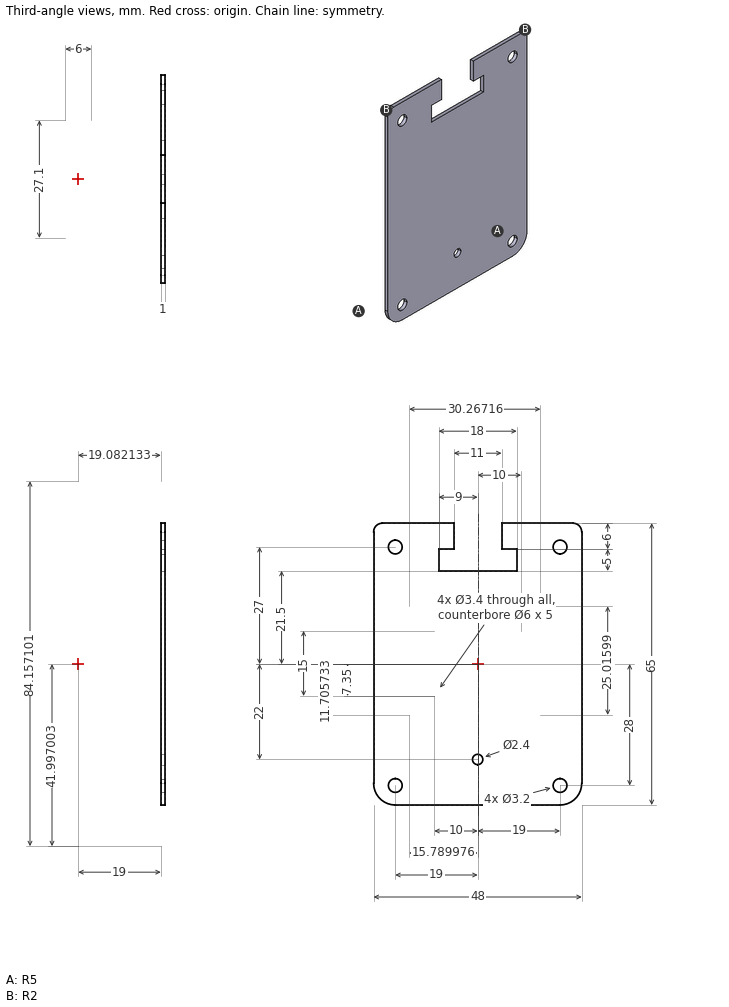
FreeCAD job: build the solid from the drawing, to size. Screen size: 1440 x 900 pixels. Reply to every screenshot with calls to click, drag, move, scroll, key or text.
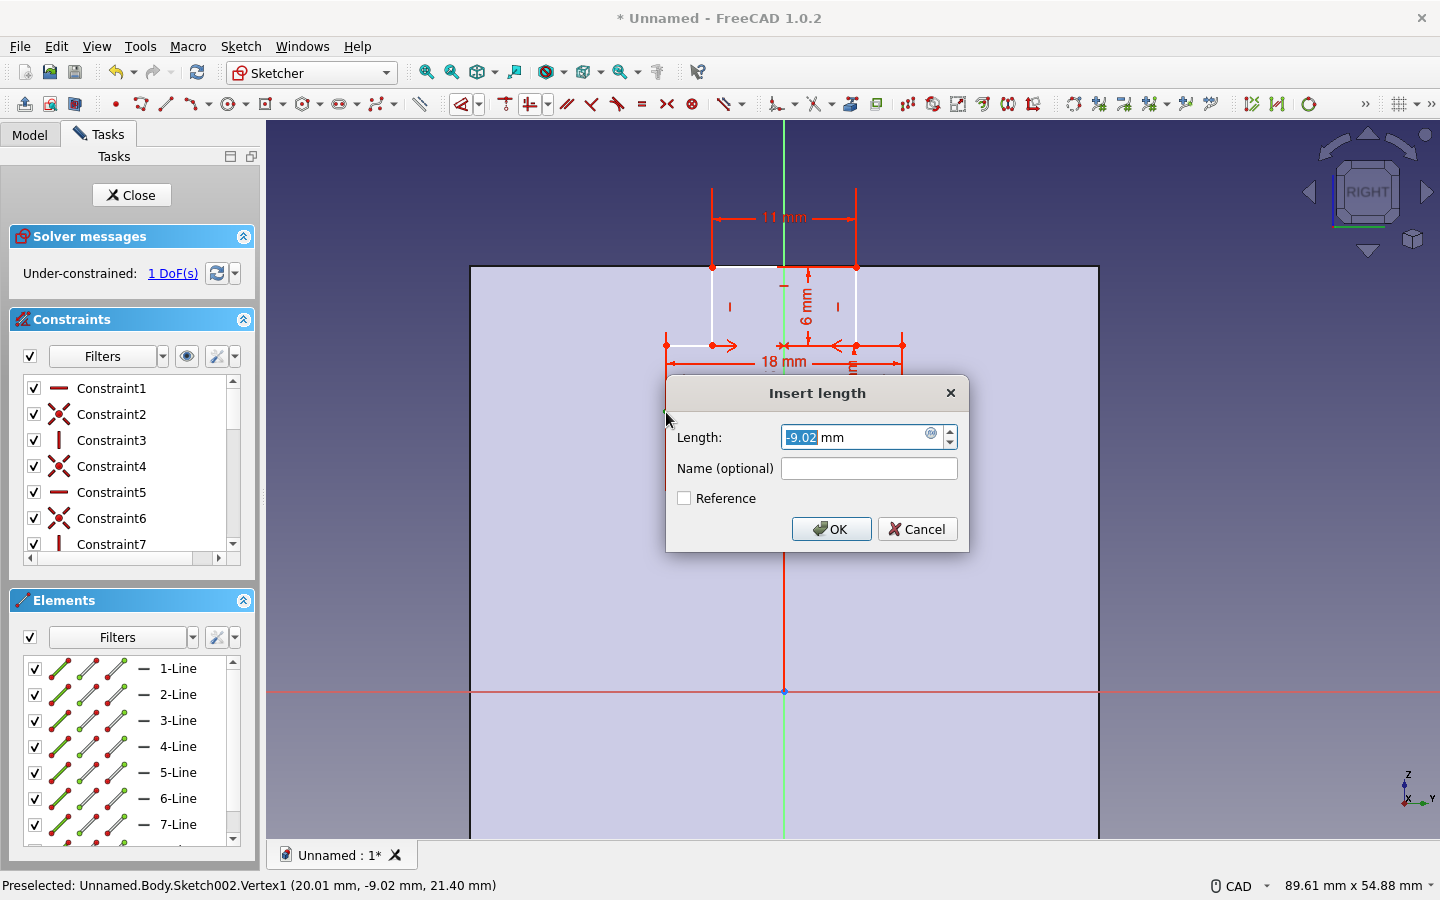
text(-9)
key(Return)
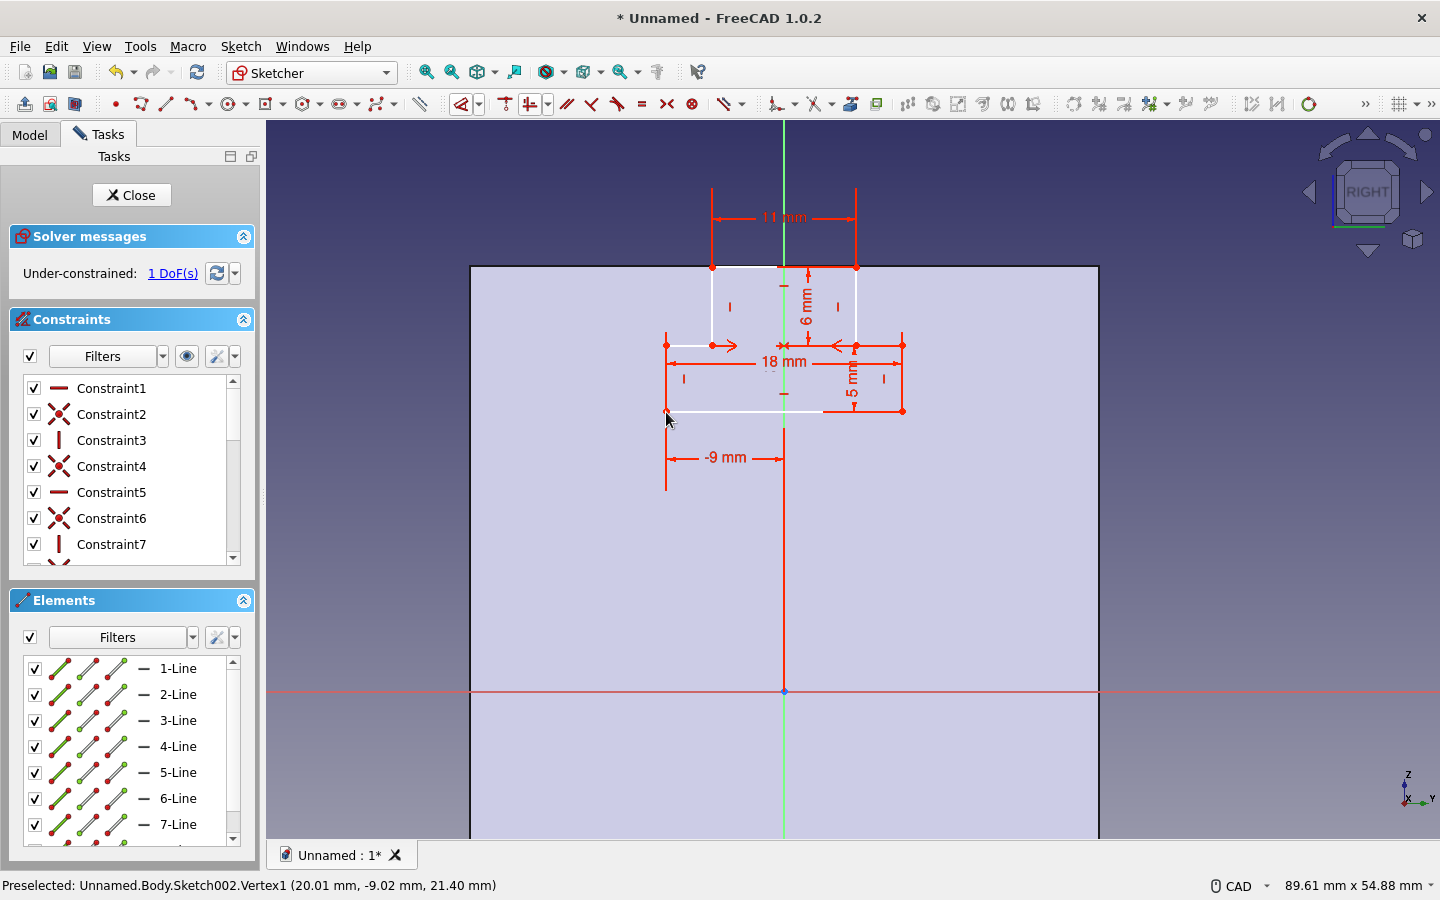
click(666, 412)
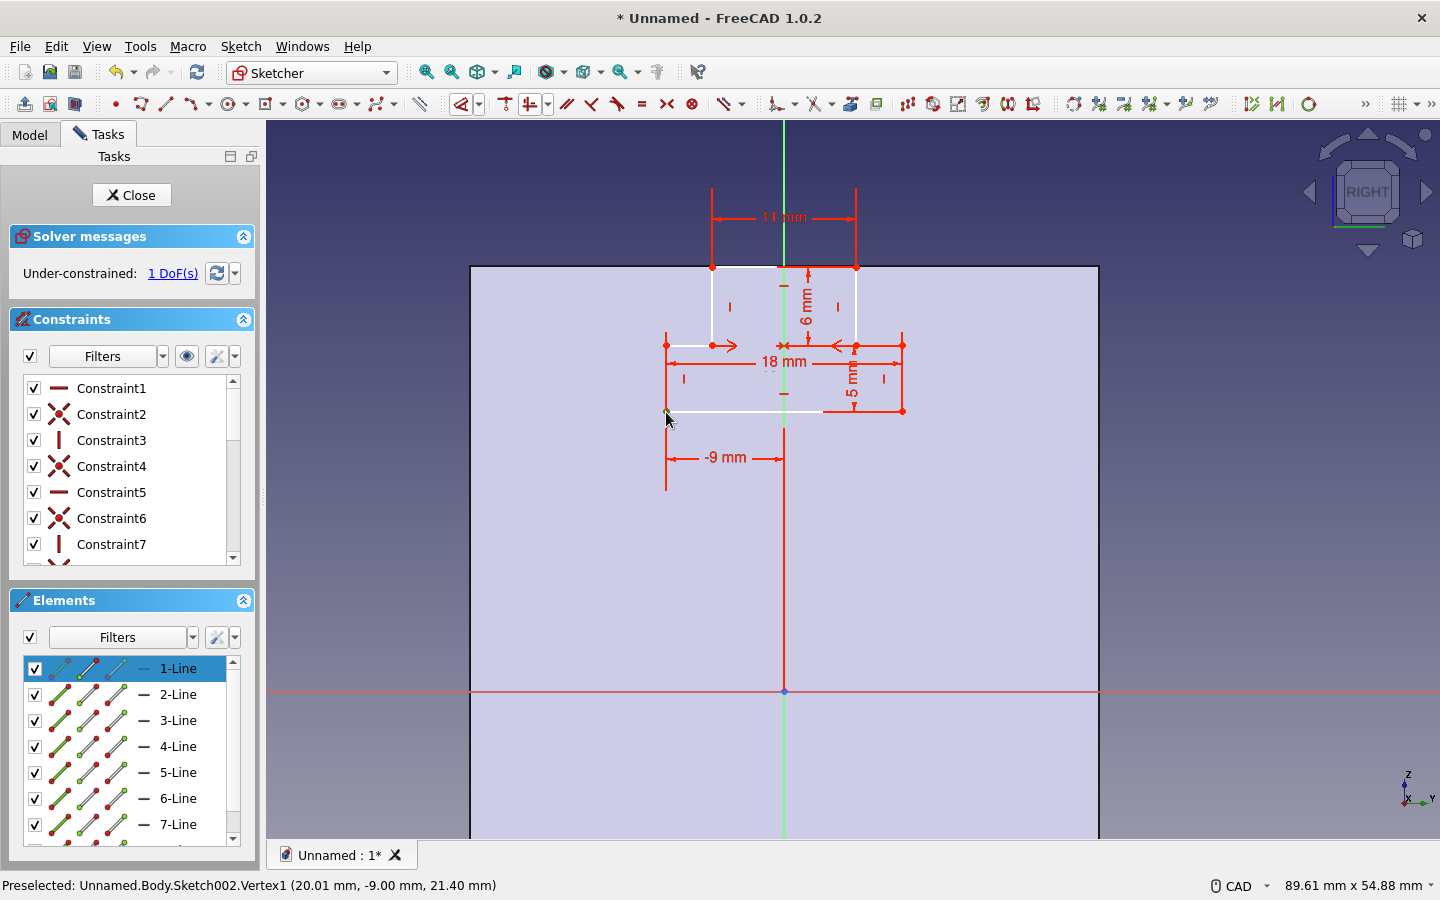
key(i)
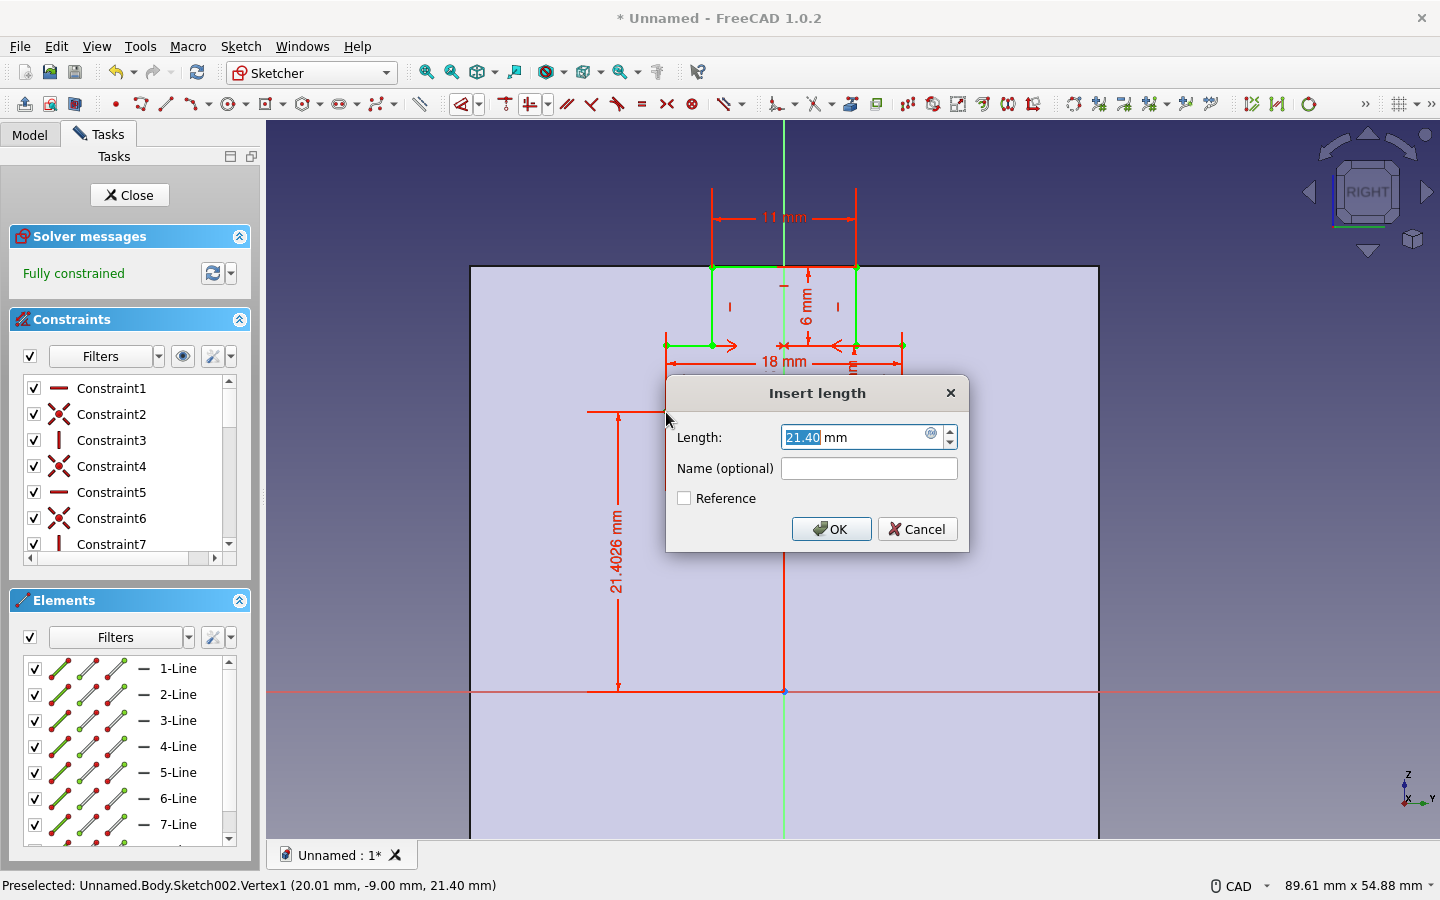
text(21.5)
key(Return)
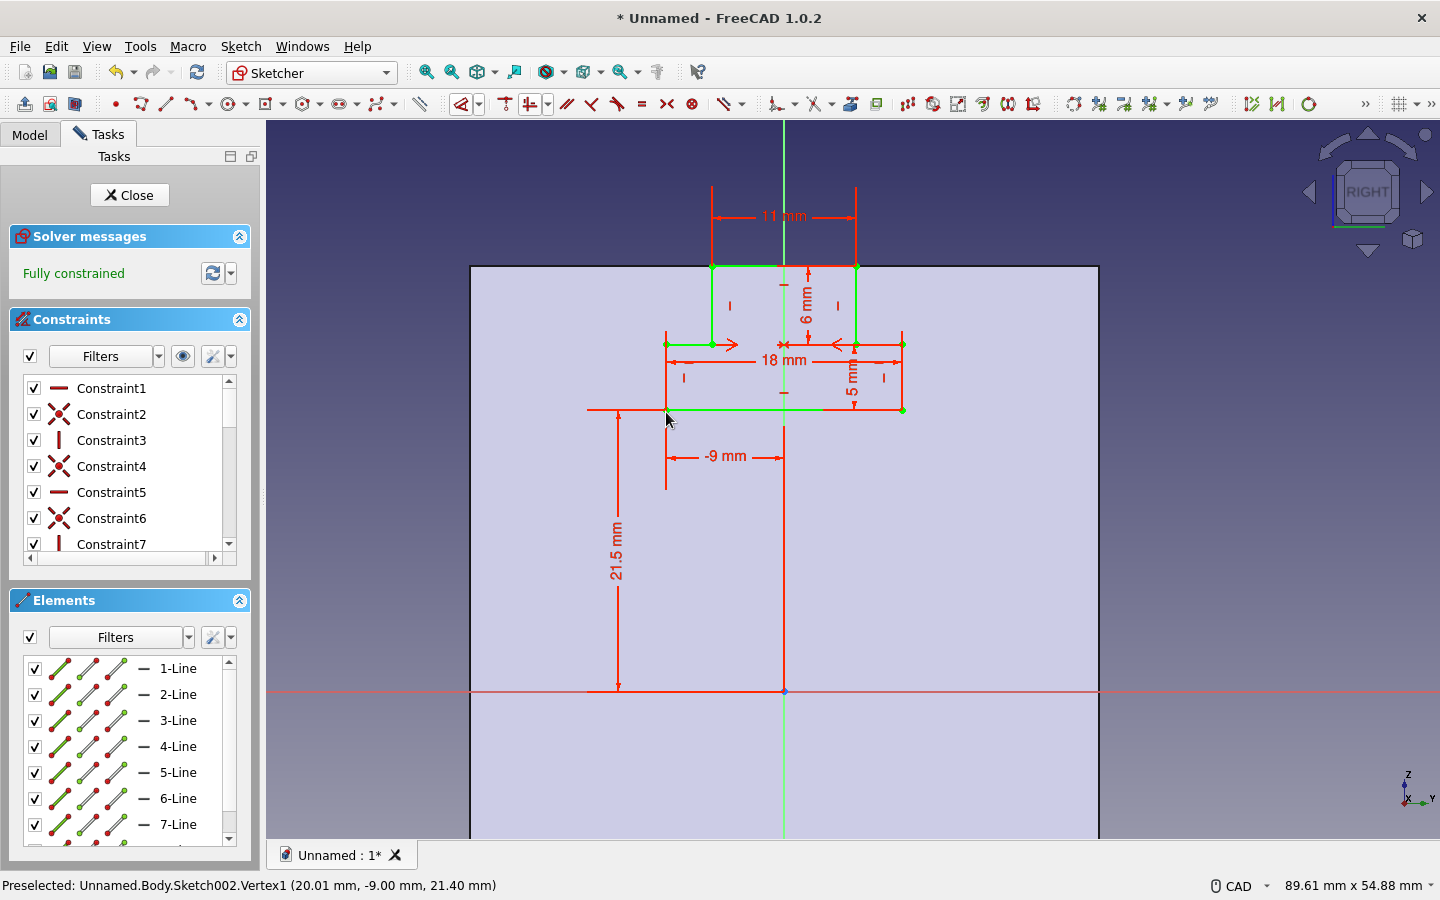
click(130, 195)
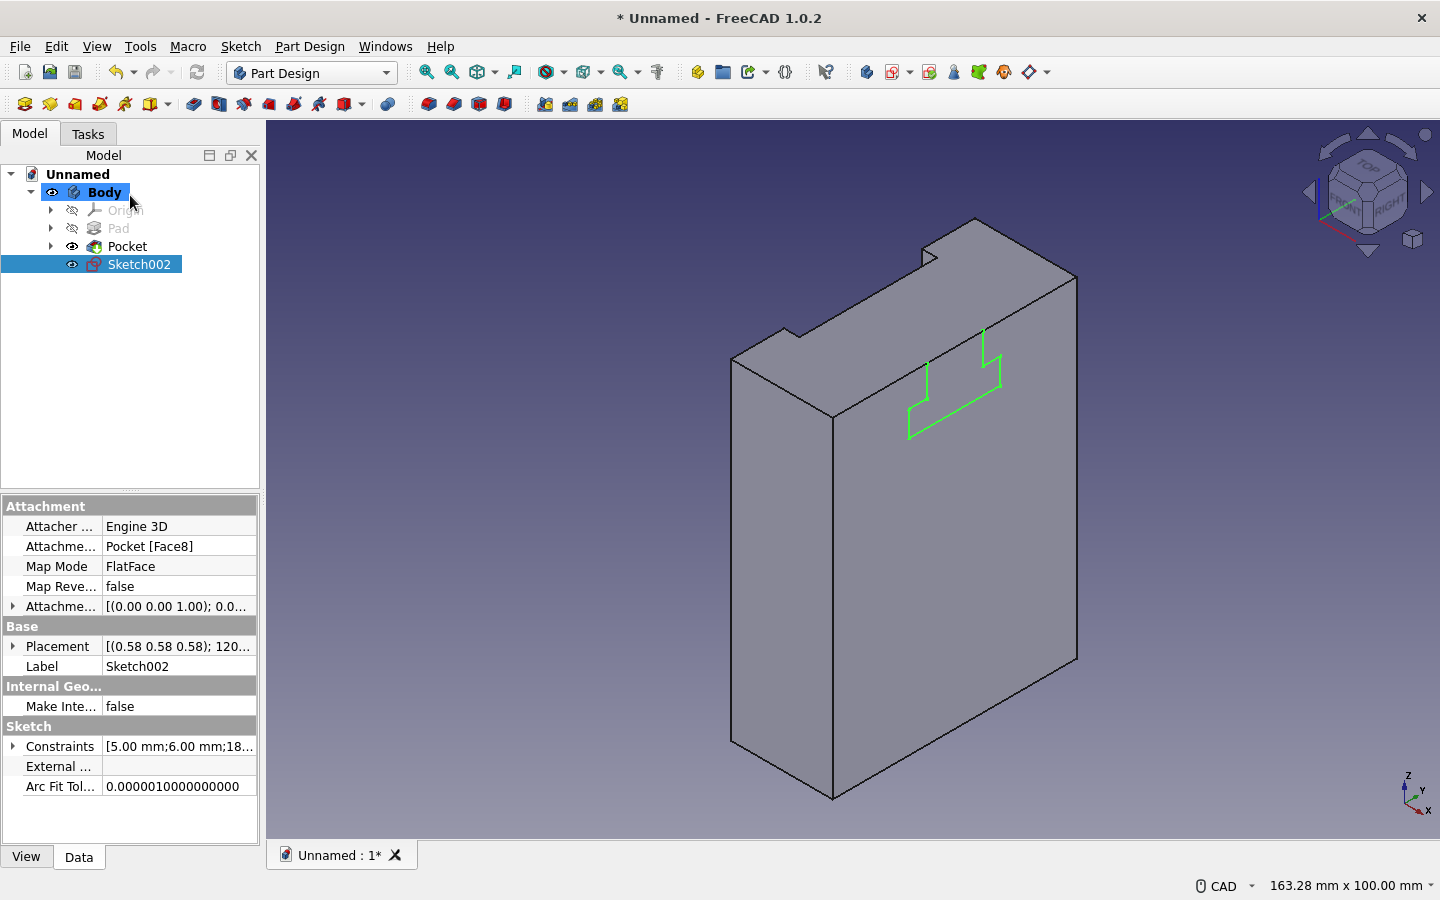
click(194, 104)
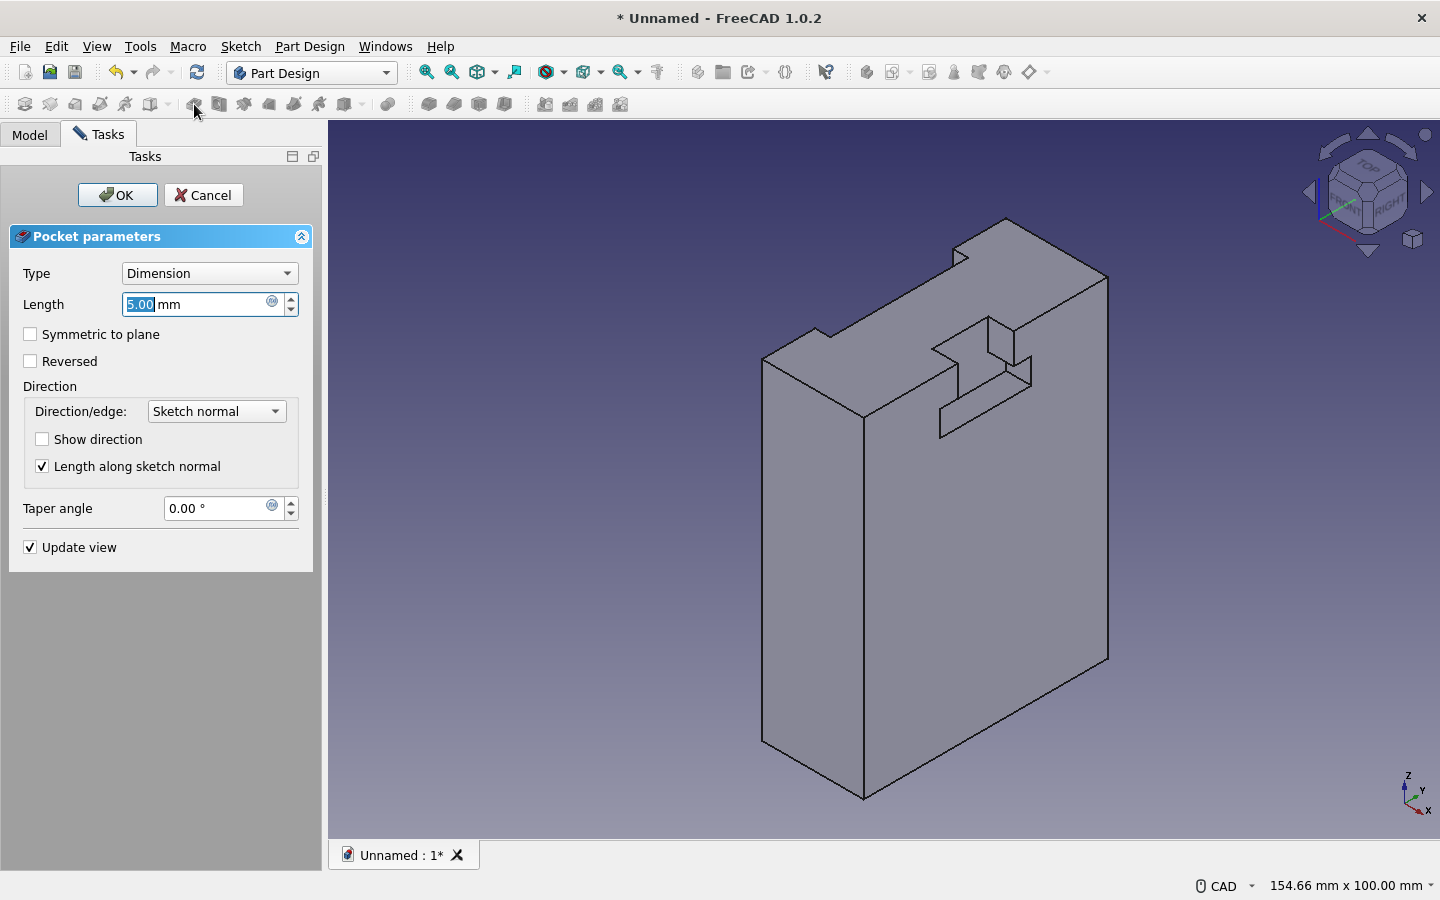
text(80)
key(Tab)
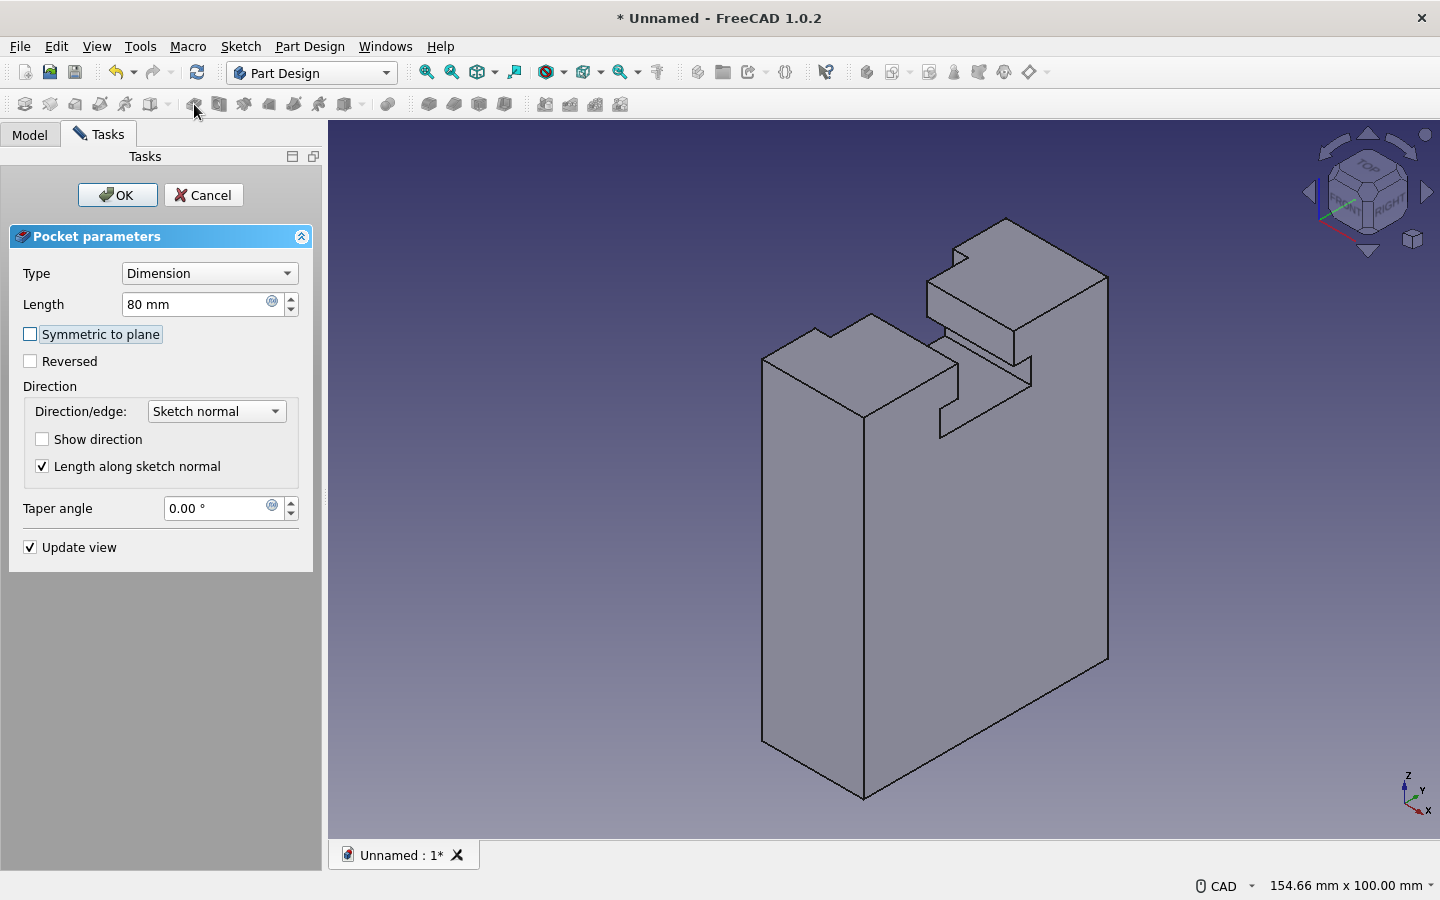
click(118, 195)